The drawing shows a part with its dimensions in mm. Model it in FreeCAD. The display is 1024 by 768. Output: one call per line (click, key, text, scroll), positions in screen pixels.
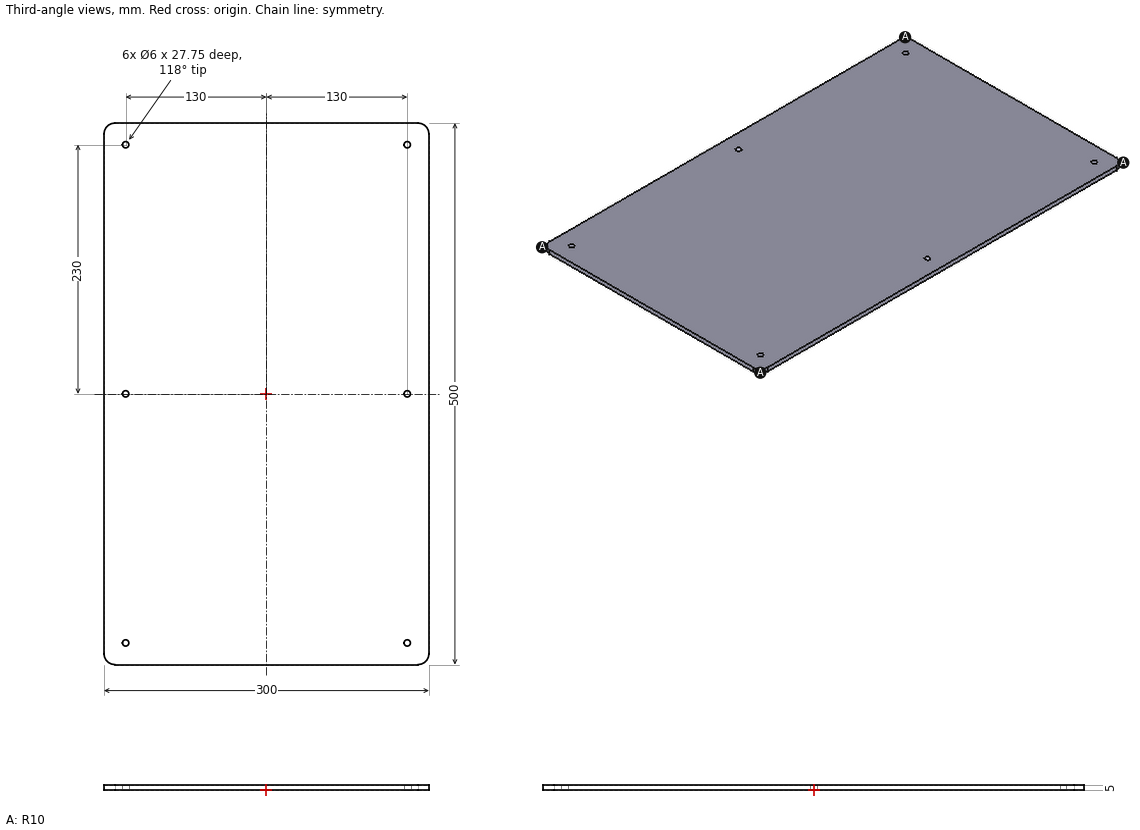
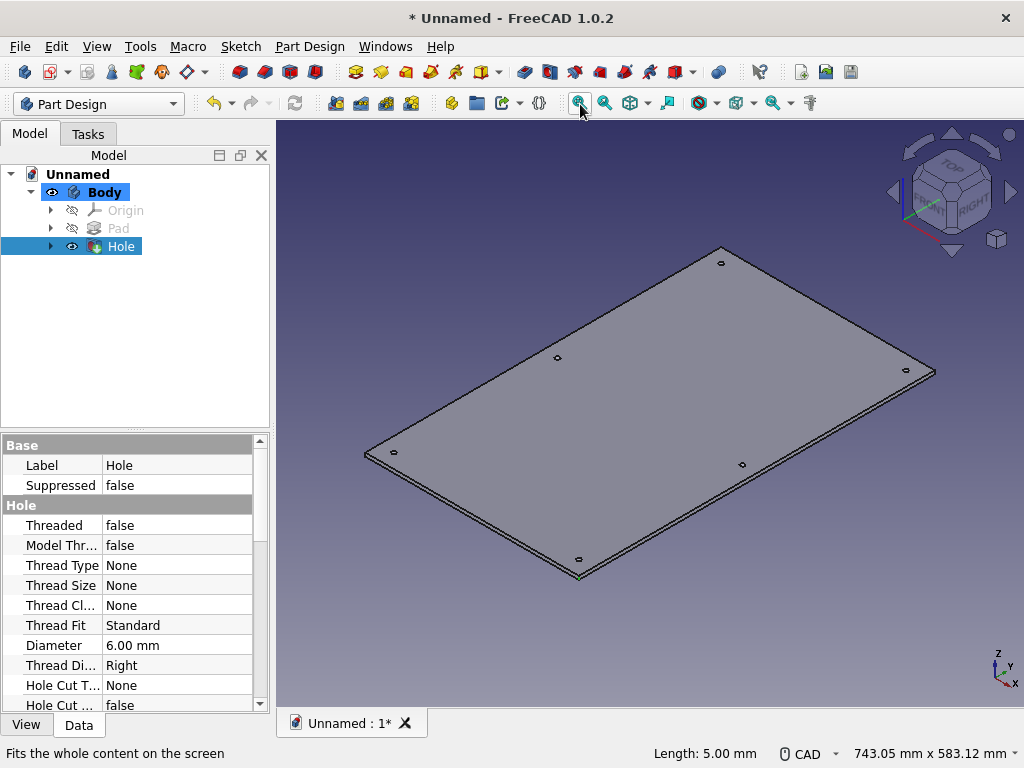
key(2)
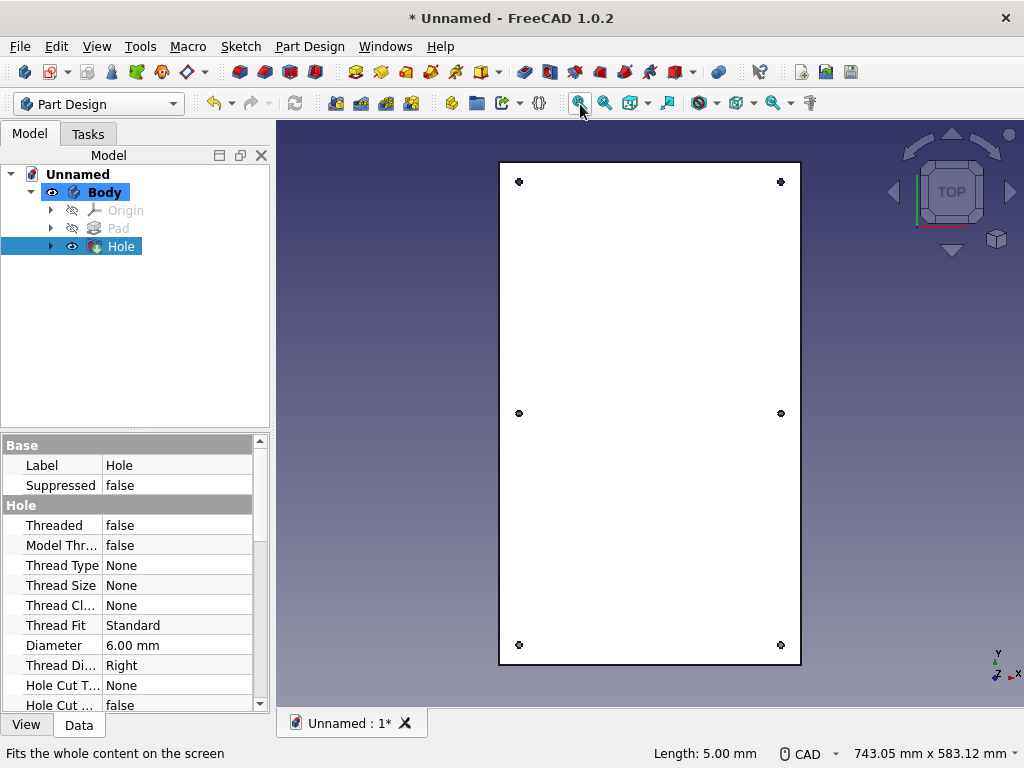
scroll(499, 664, up, 11)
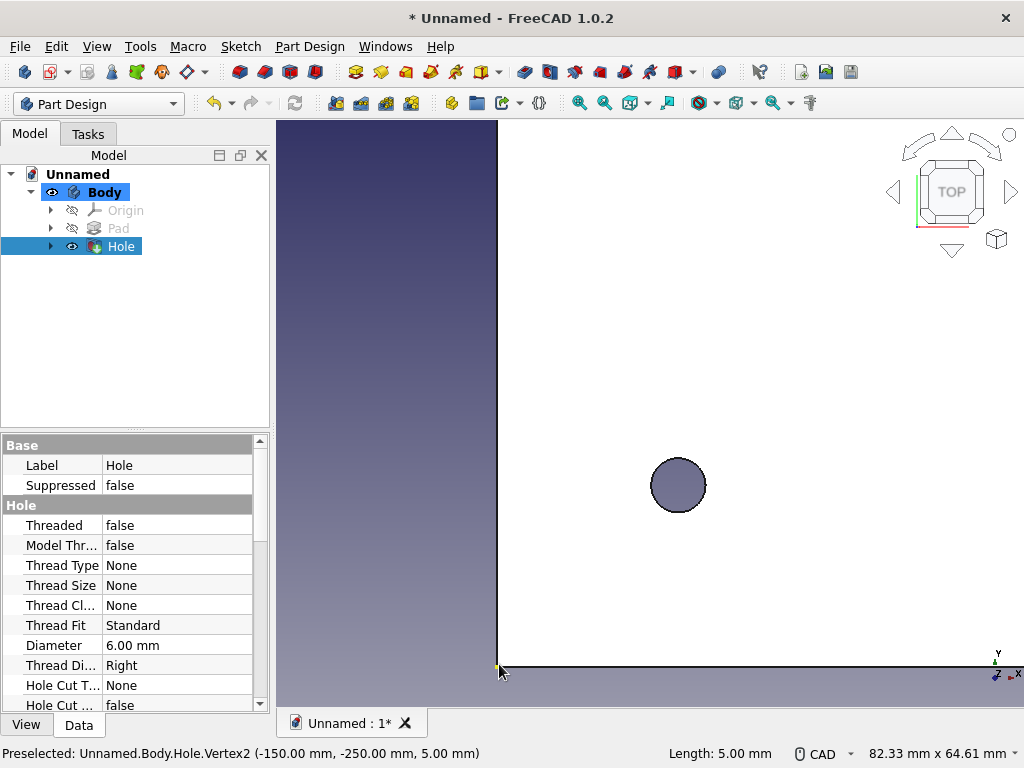
click(580, 104)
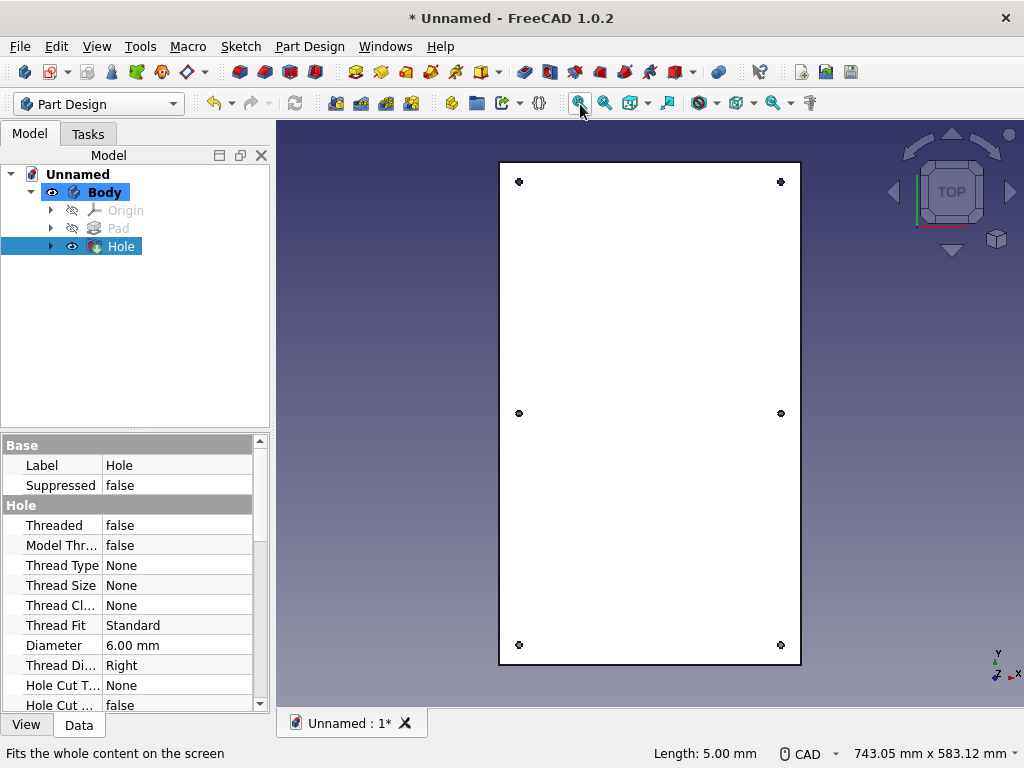
key(1)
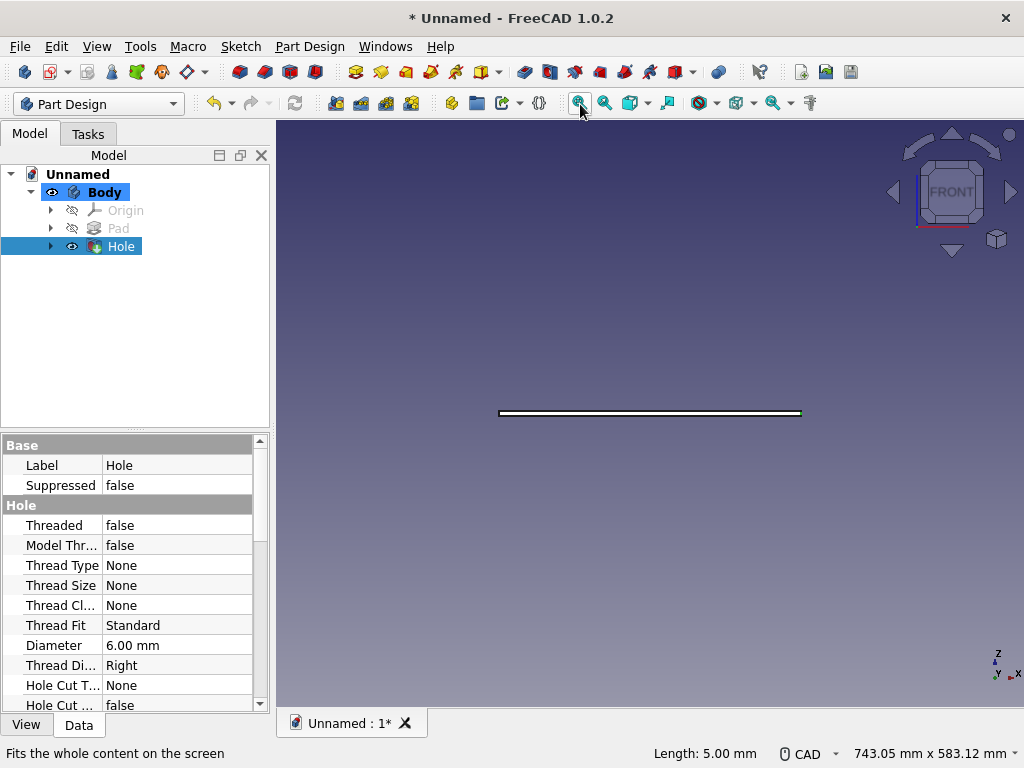
click(580, 104)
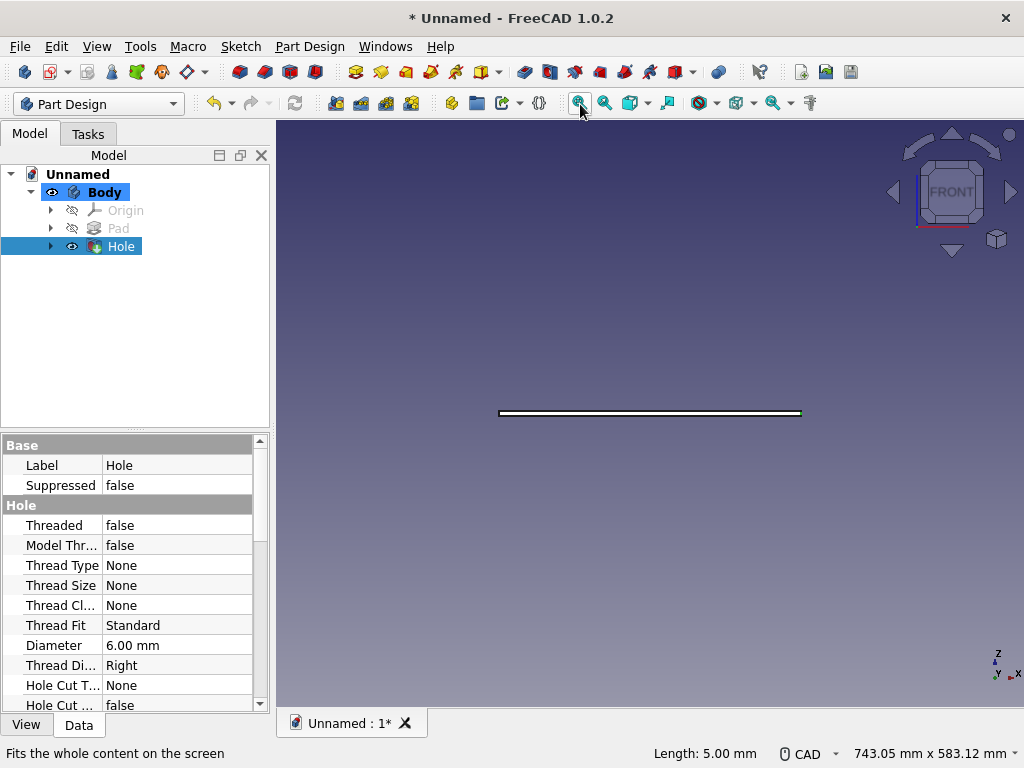
scroll(499, 413, up, 11)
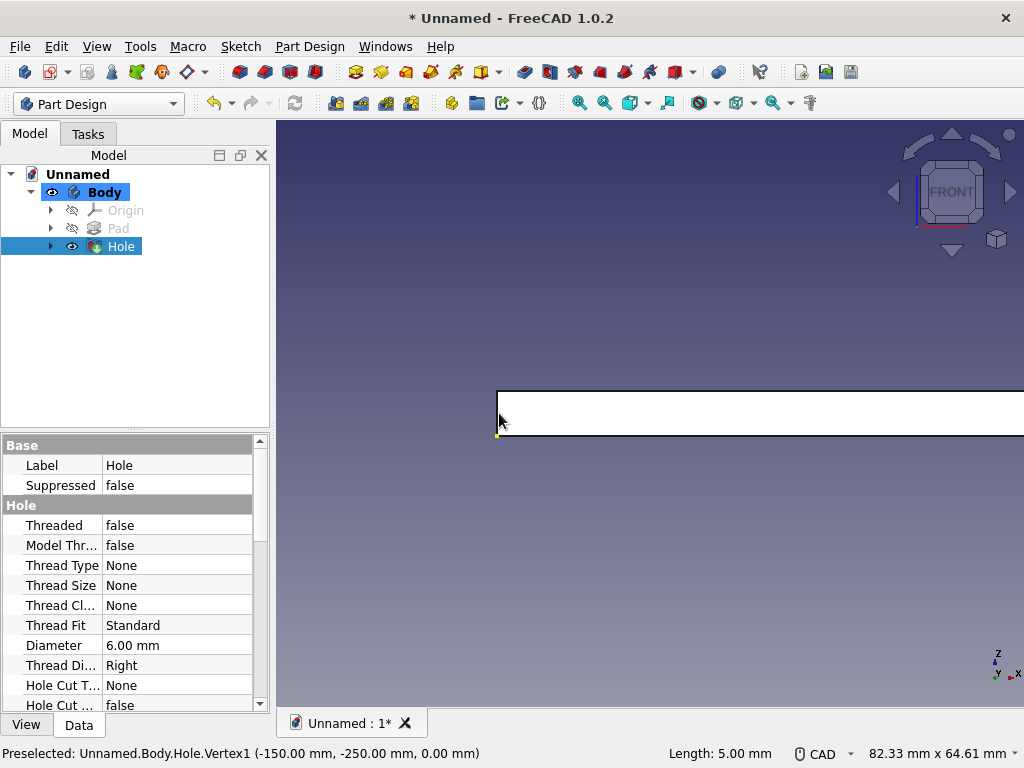
click(497, 413, ctrl)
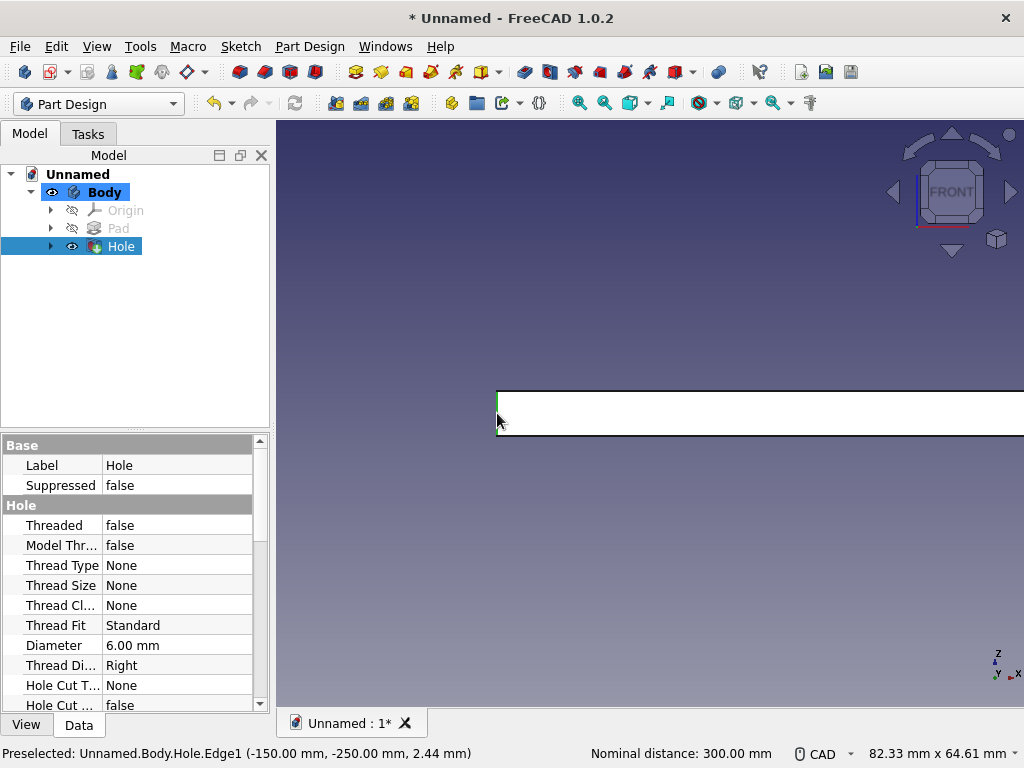
click(580, 104)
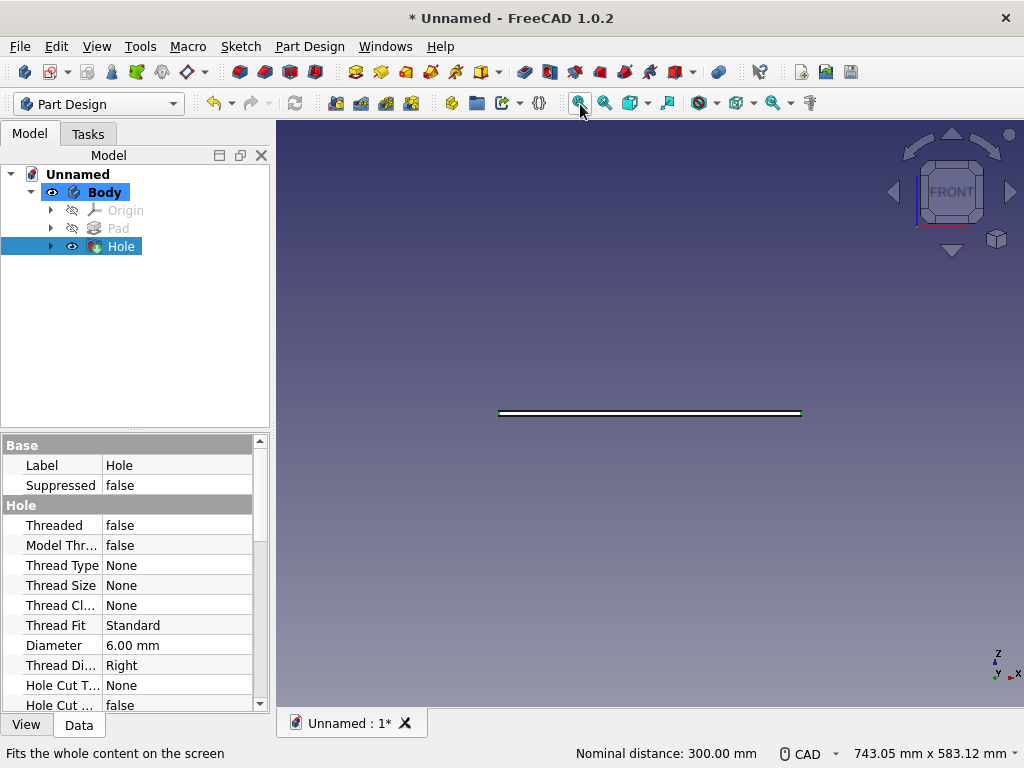
key(3)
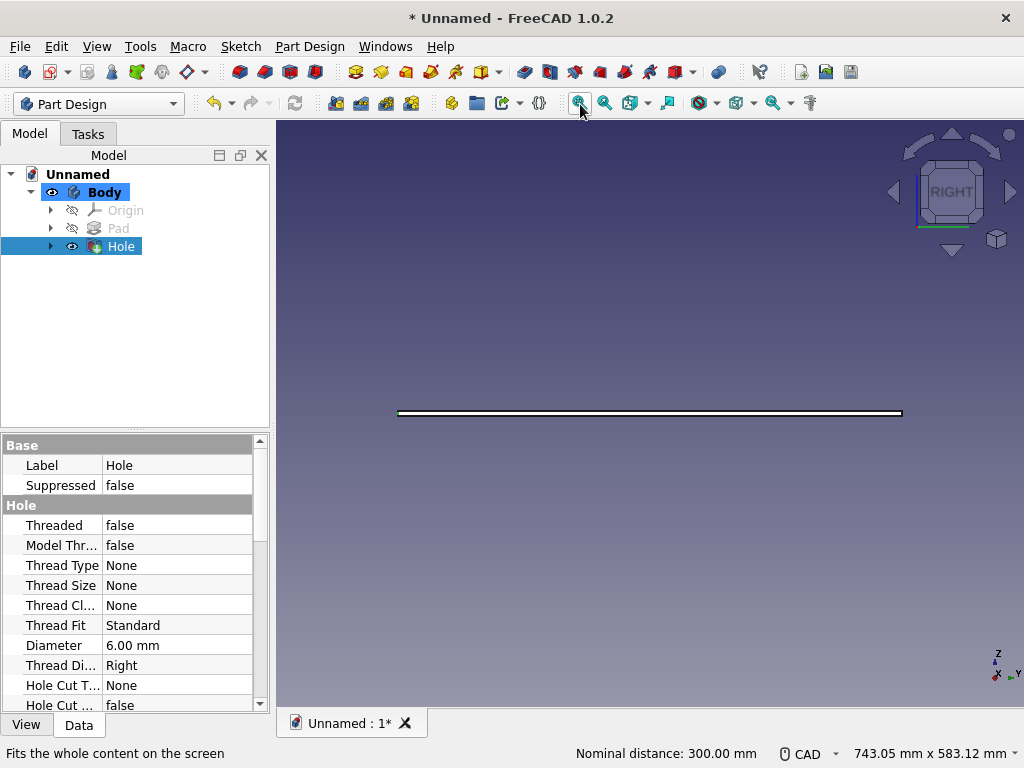
key(5)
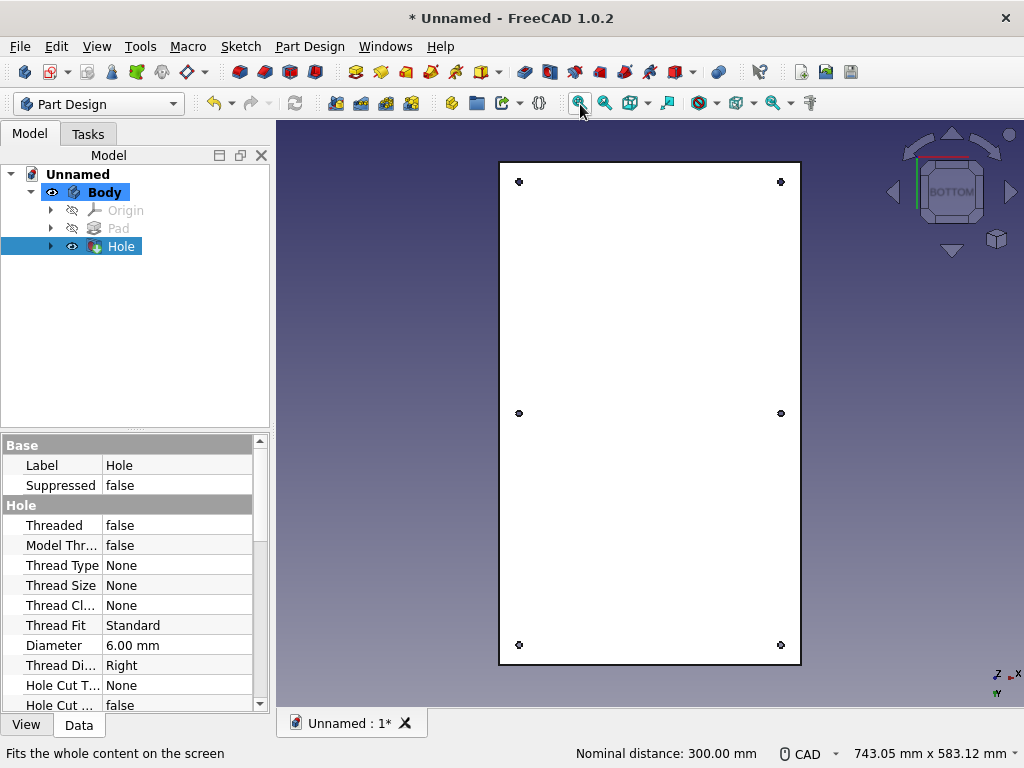
scroll(499, 664, up, 11)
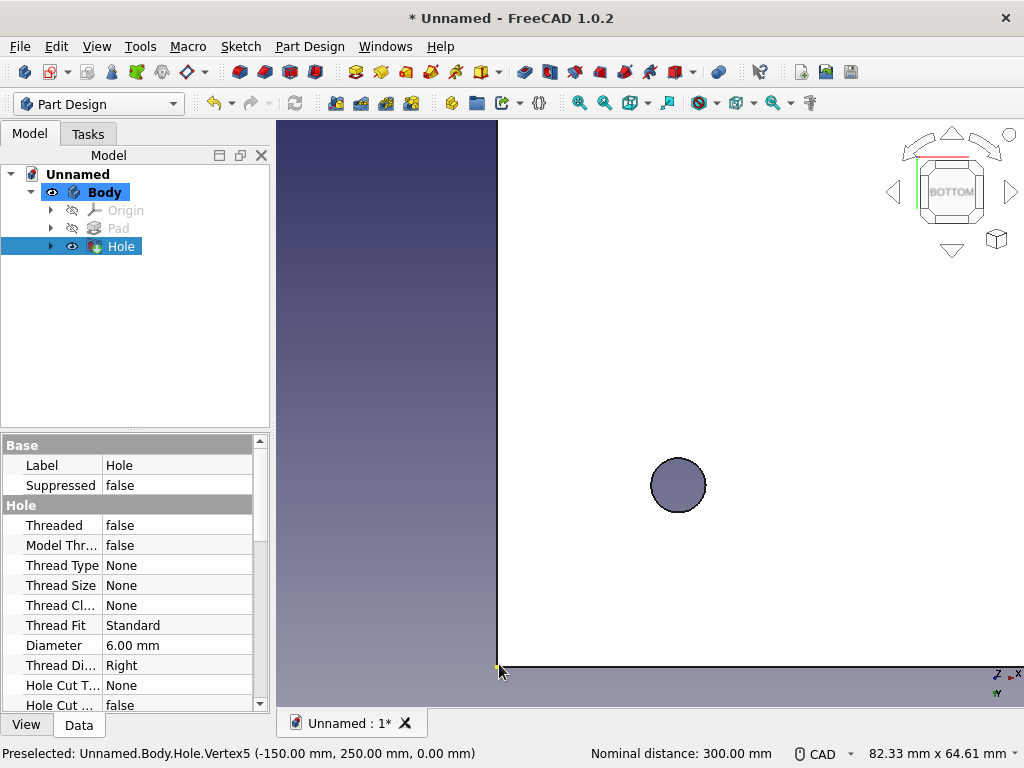
click(580, 104)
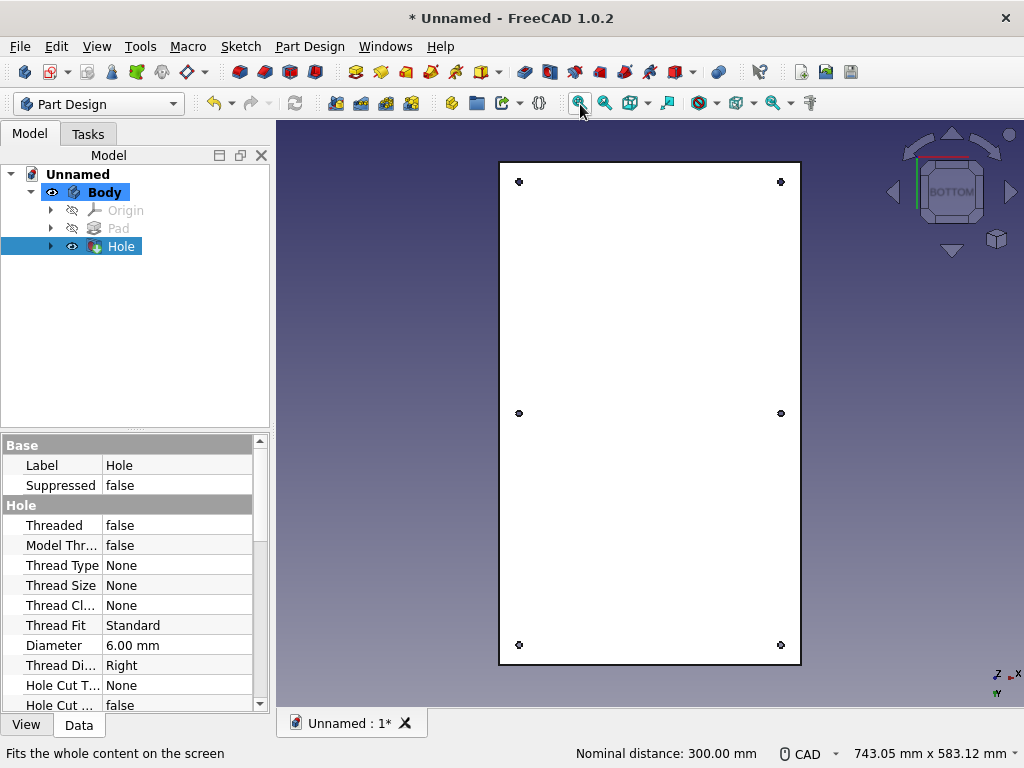
key(4)